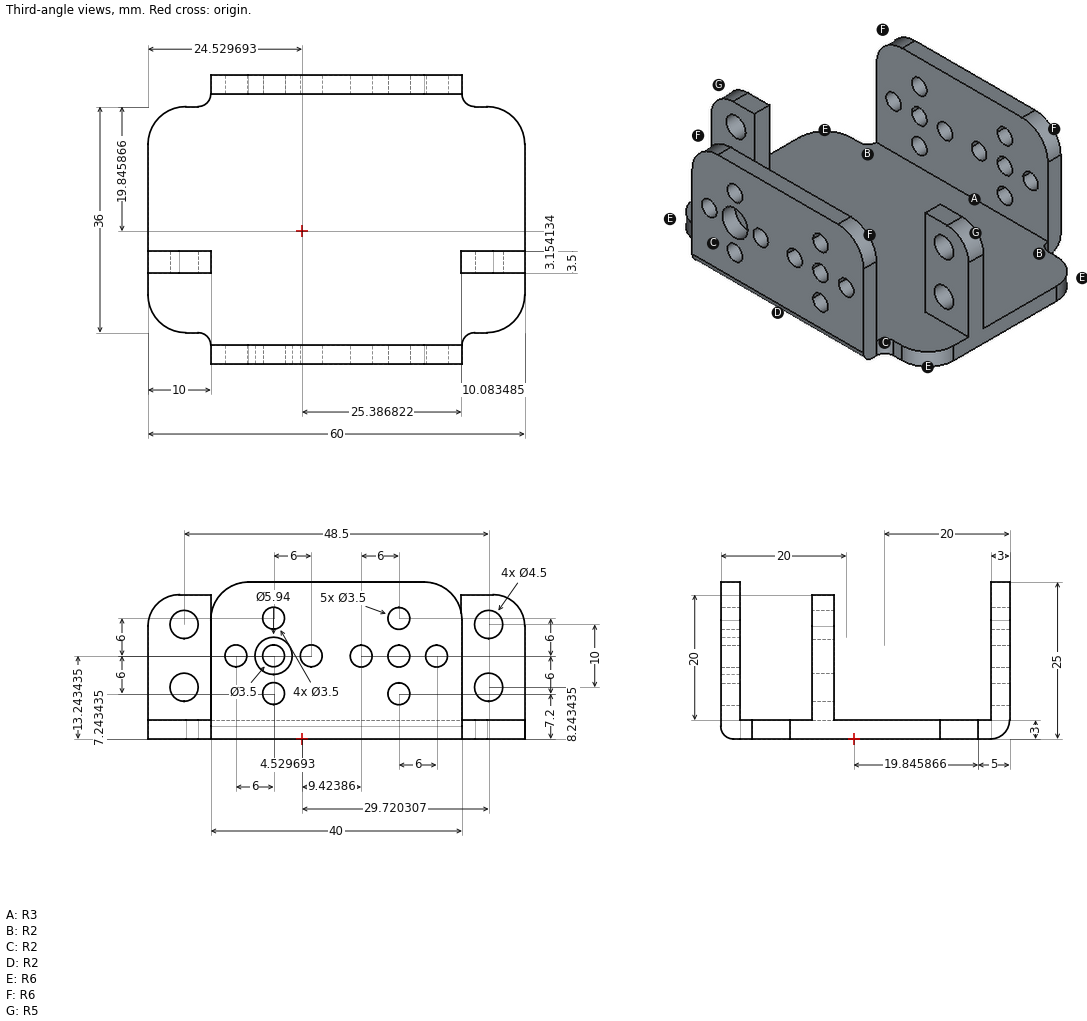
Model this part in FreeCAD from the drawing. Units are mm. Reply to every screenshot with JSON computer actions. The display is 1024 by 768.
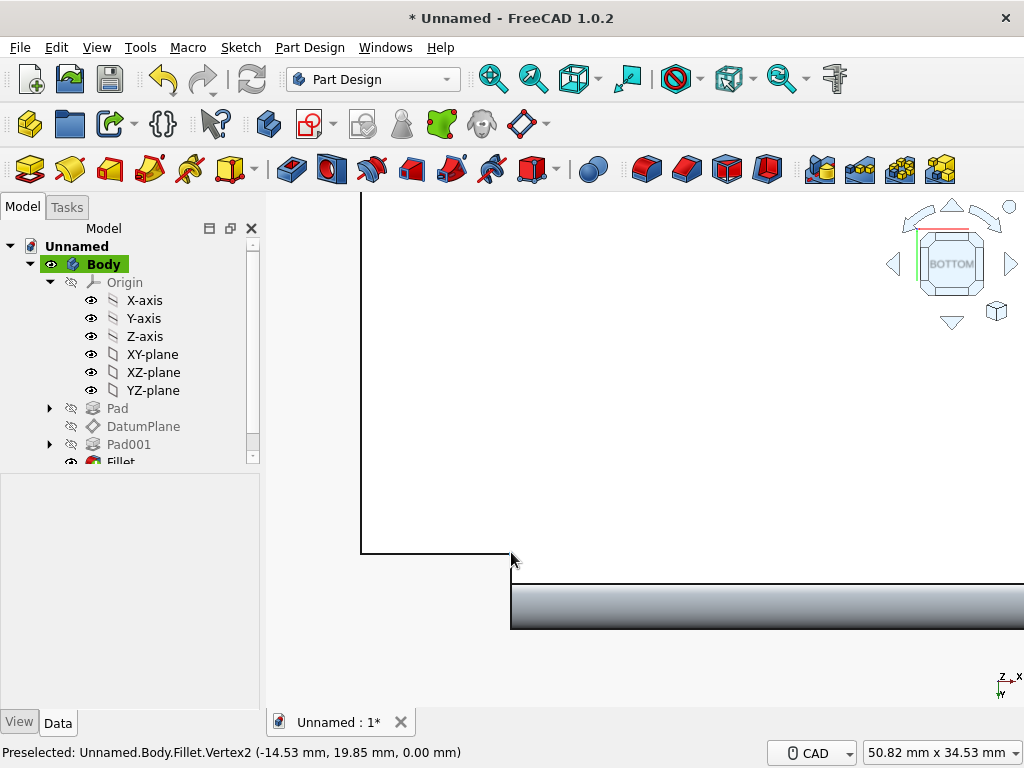
{"action": "left_click", "coordinate": [494, 80]}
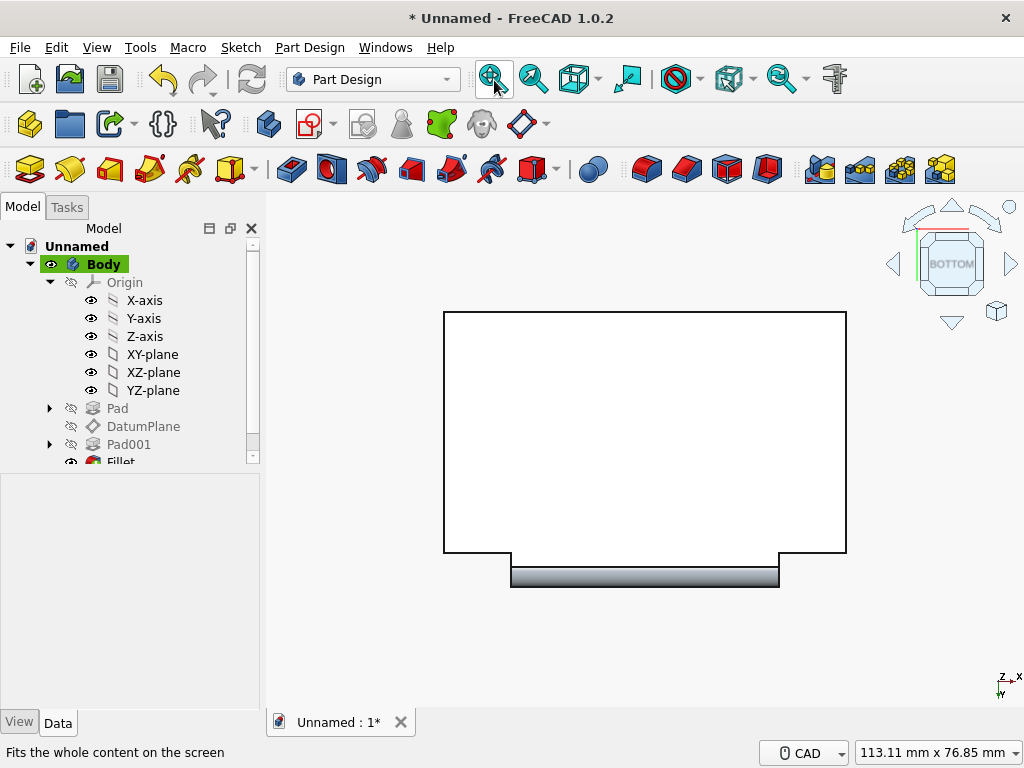
{"action": "key", "text": "4"}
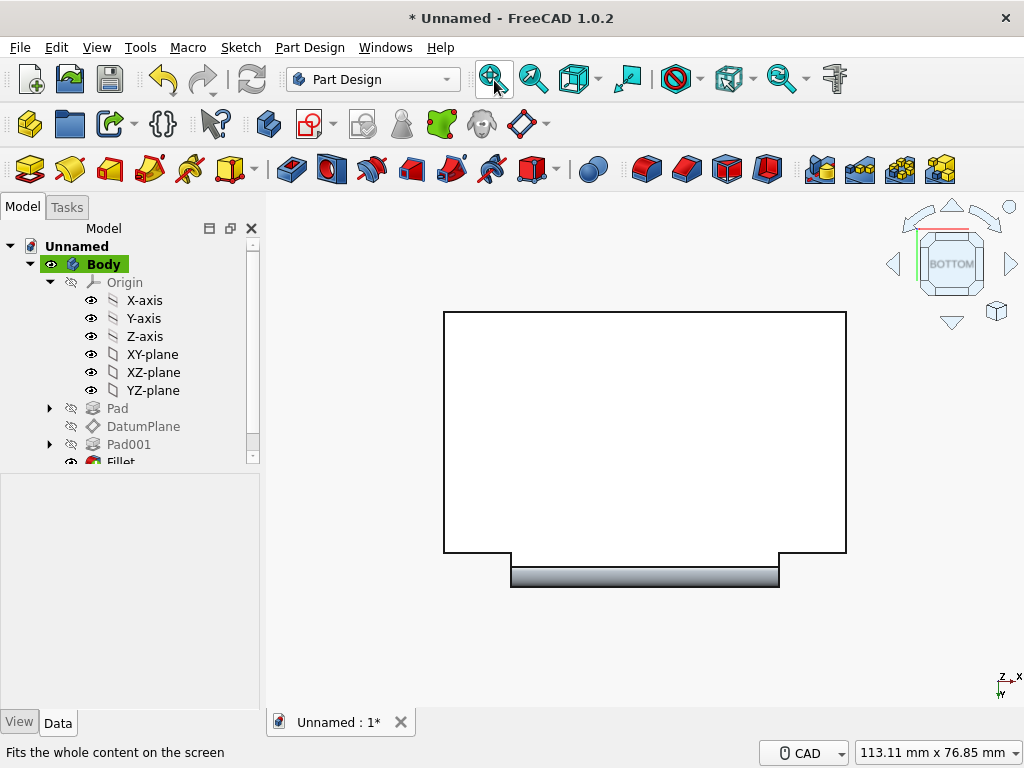
{"action": "scroll", "coordinate": [779, 522], "scroll_direction": "up", "scroll_amount": 4}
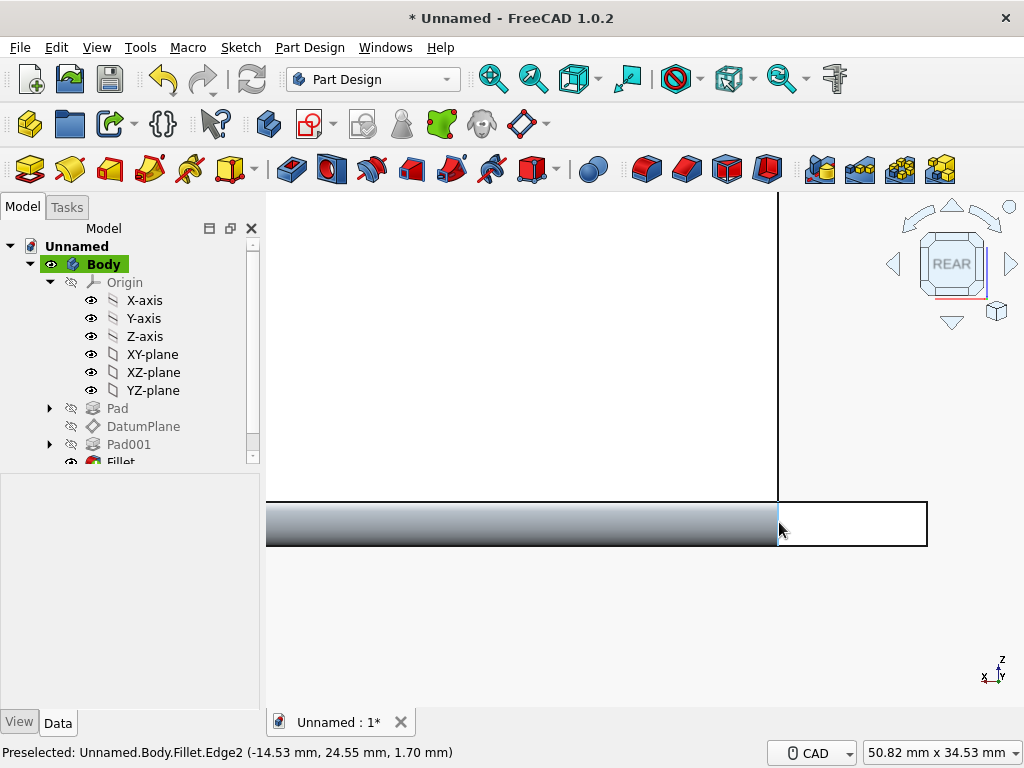
{"action": "left_click", "coordinate": [494, 80]}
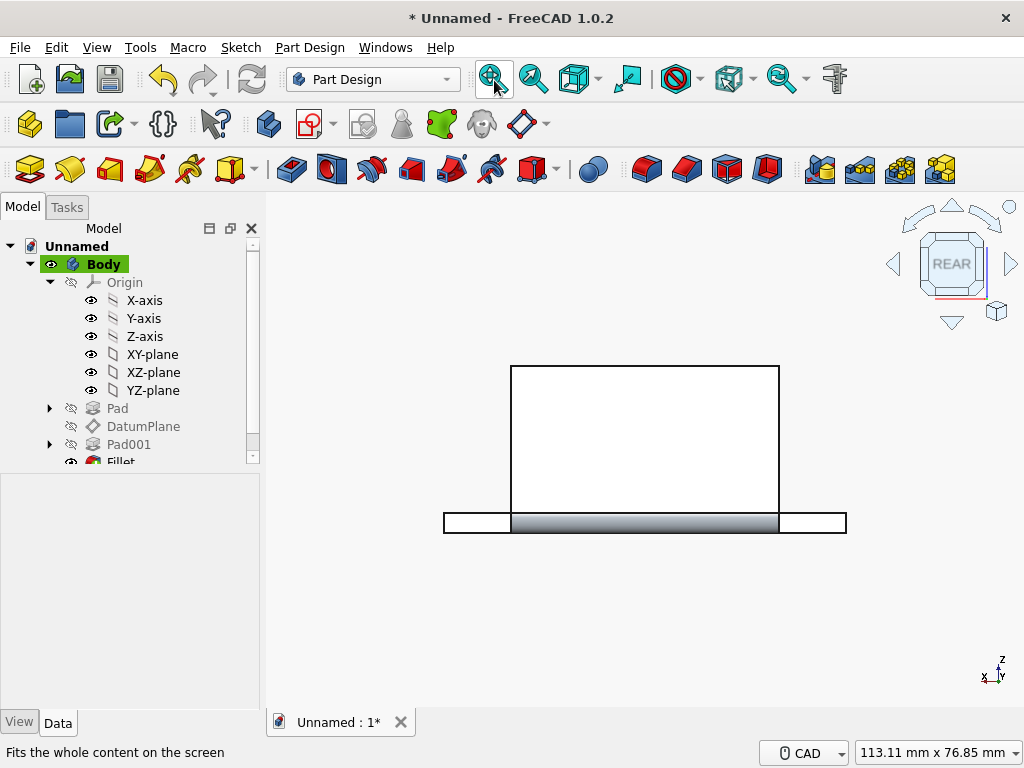
{"action": "key", "text": "6"}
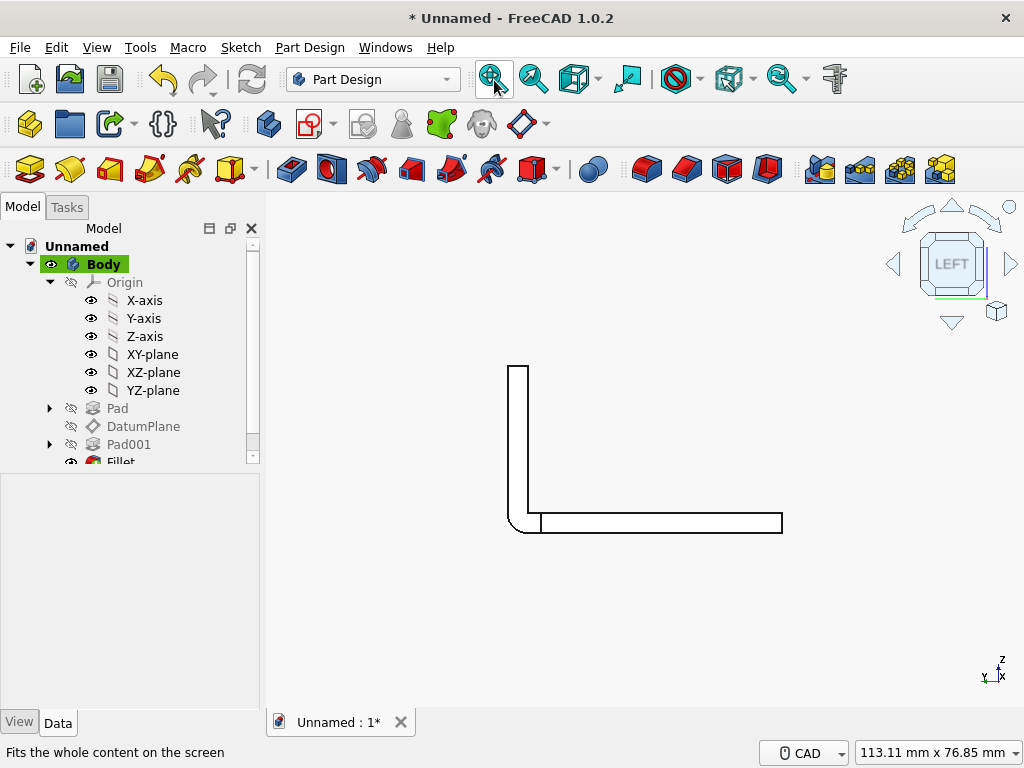
{"action": "left_click", "coordinate": [494, 80]}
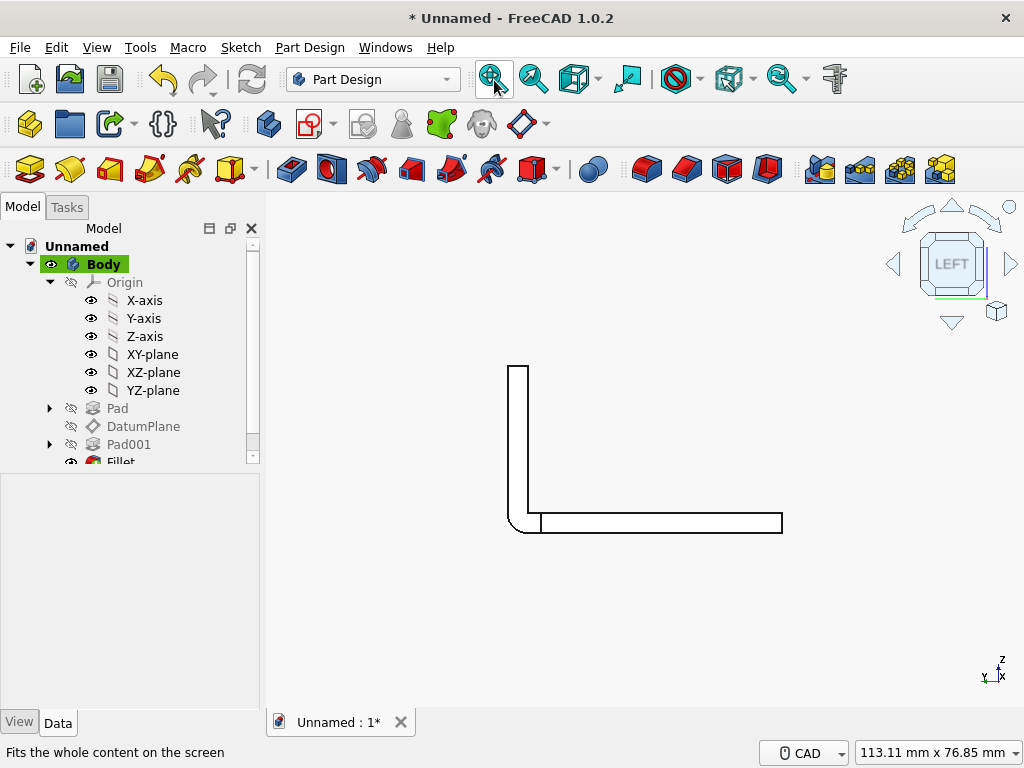
{"action": "scroll", "coordinate": [541, 522], "scroll_direction": "up", "scroll_amount": 4}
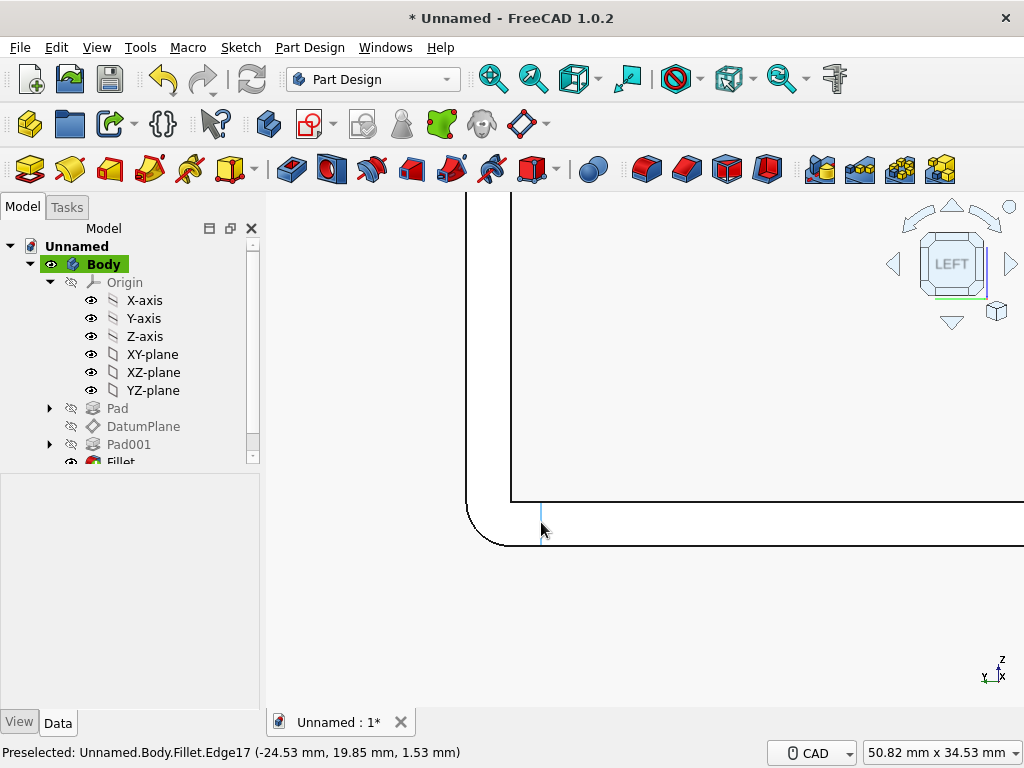
{"action": "left_click", "coordinate": [494, 80]}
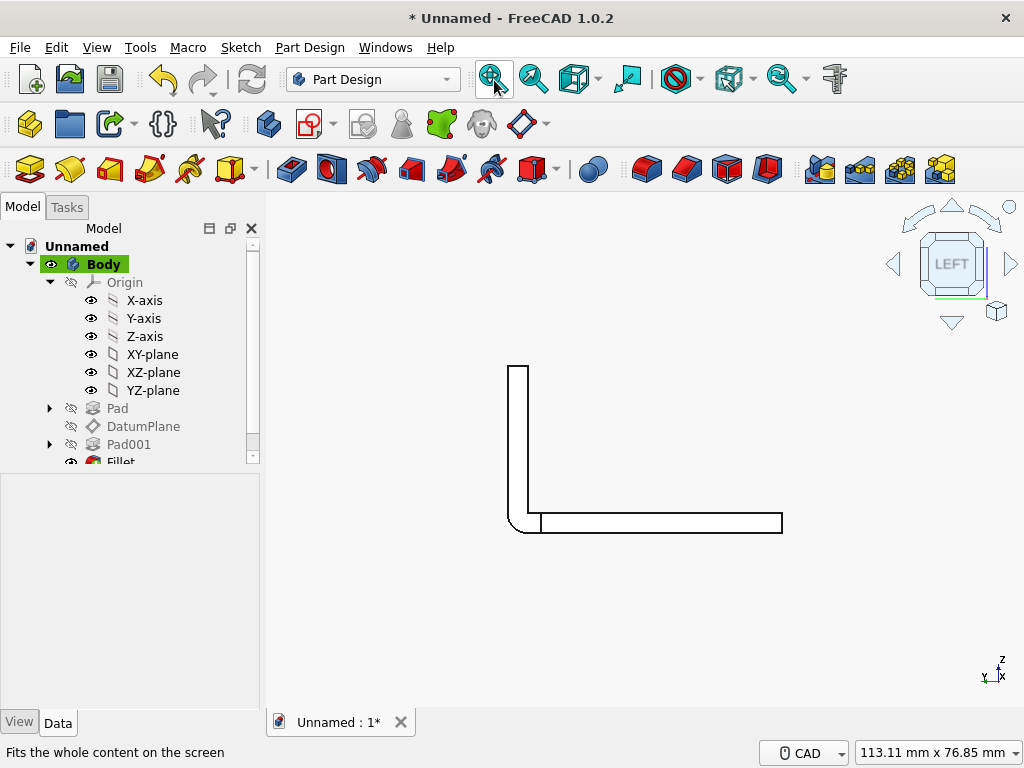
{"action": "key", "text": "v 3"}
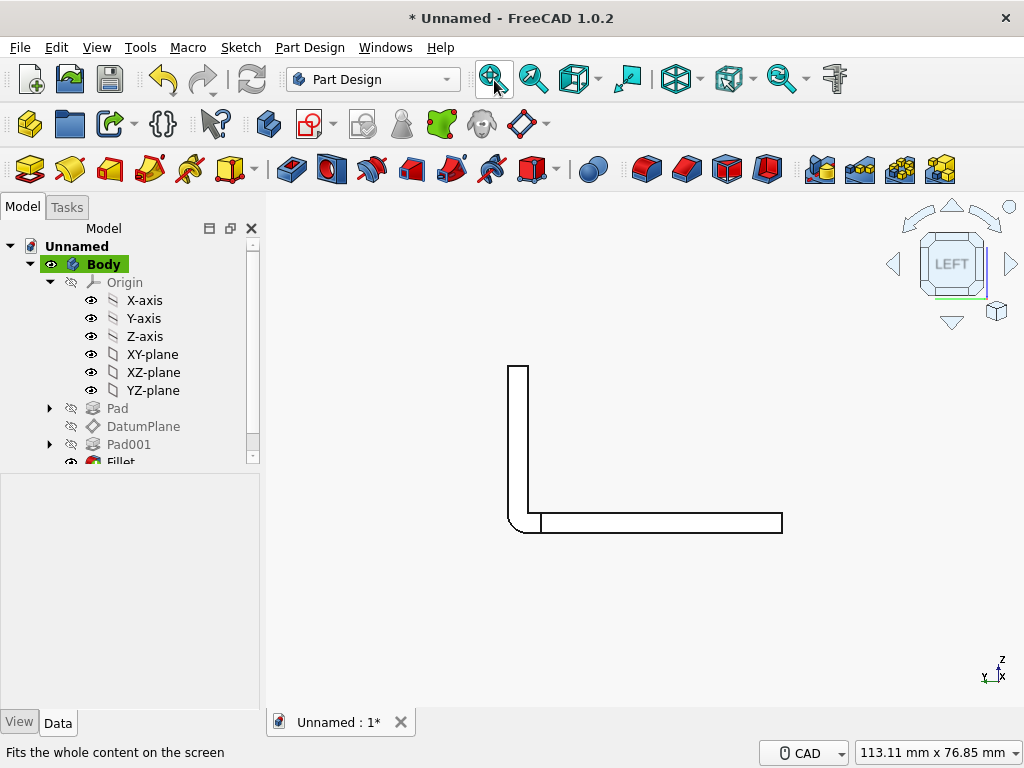
{"action": "key", "text": "0"}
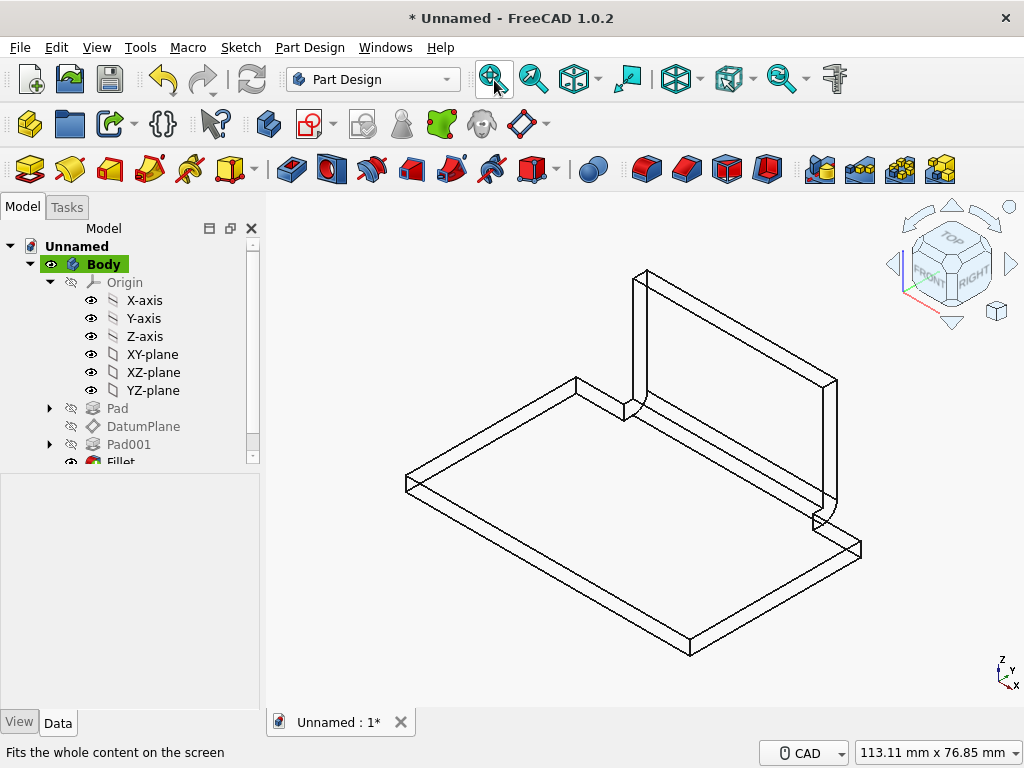
{"action": "left_click", "coordinate": [624, 412]}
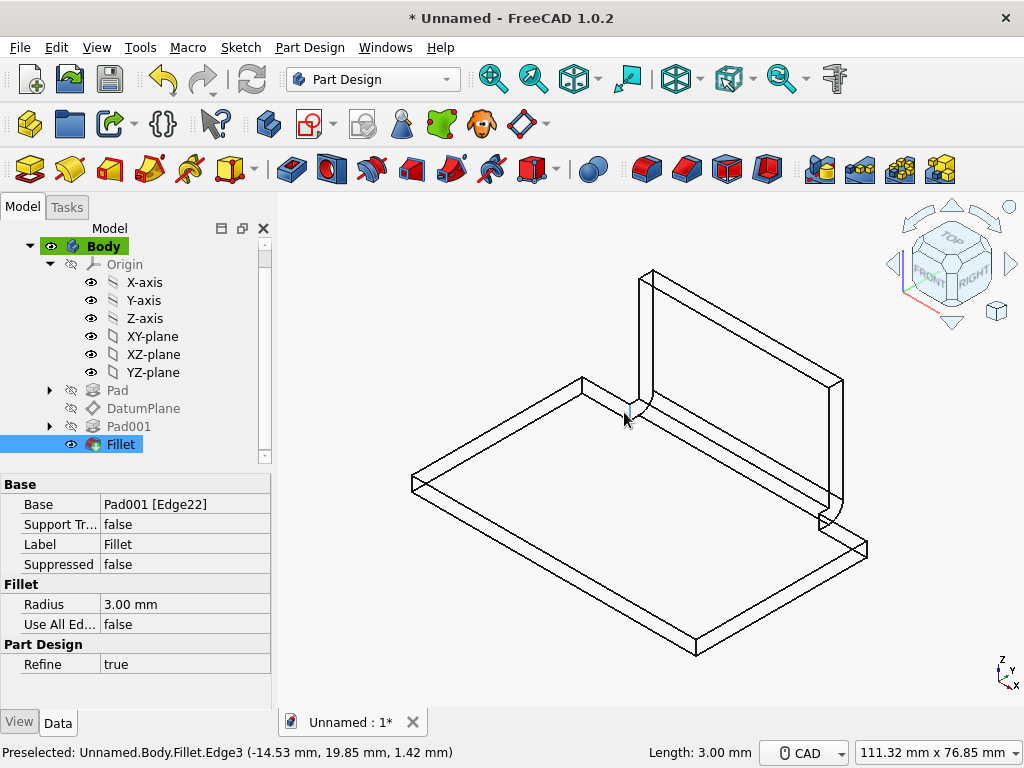
{"action": "left_click", "coordinate": [819, 521], "text": "ctrl"}